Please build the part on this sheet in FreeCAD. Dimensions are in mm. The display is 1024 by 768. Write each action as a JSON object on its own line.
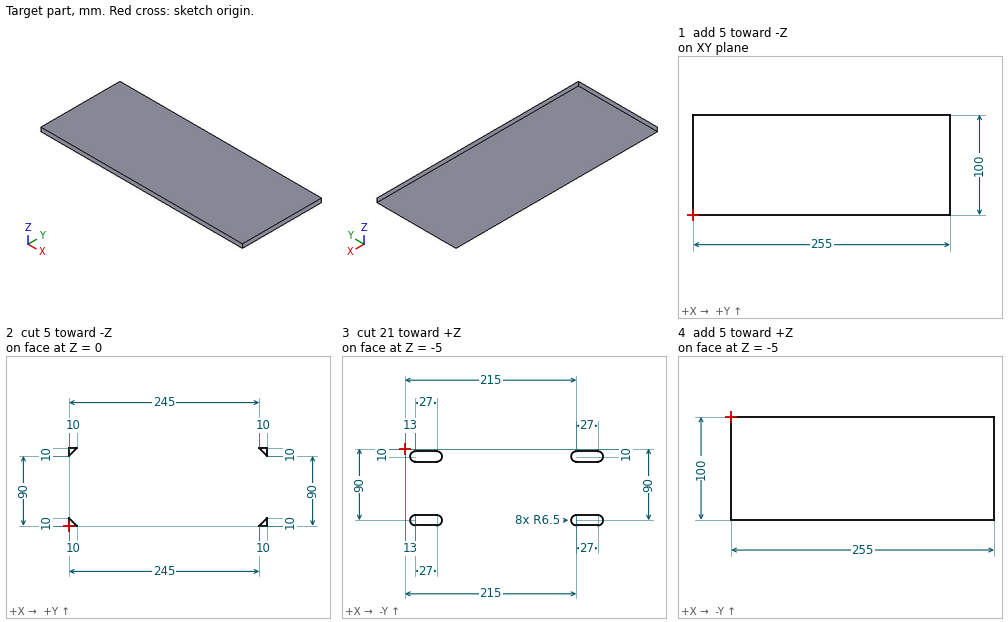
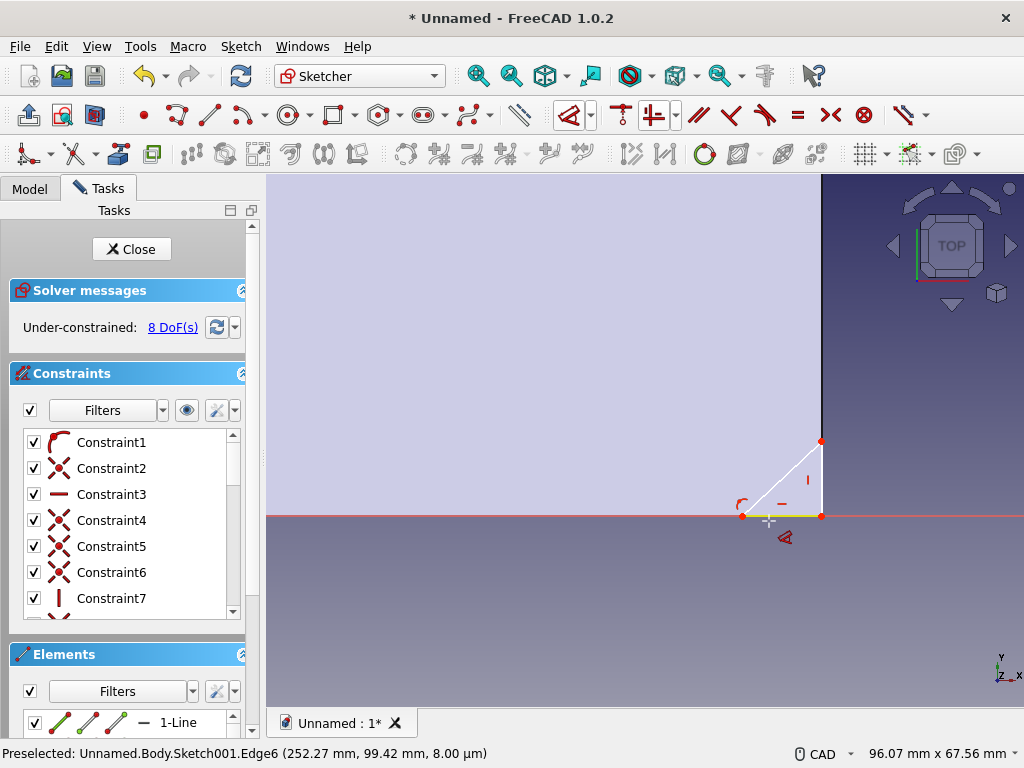
{"action": "left_click", "coordinate": [766, 516]}
{"action": "left_click", "coordinate": [782, 550]}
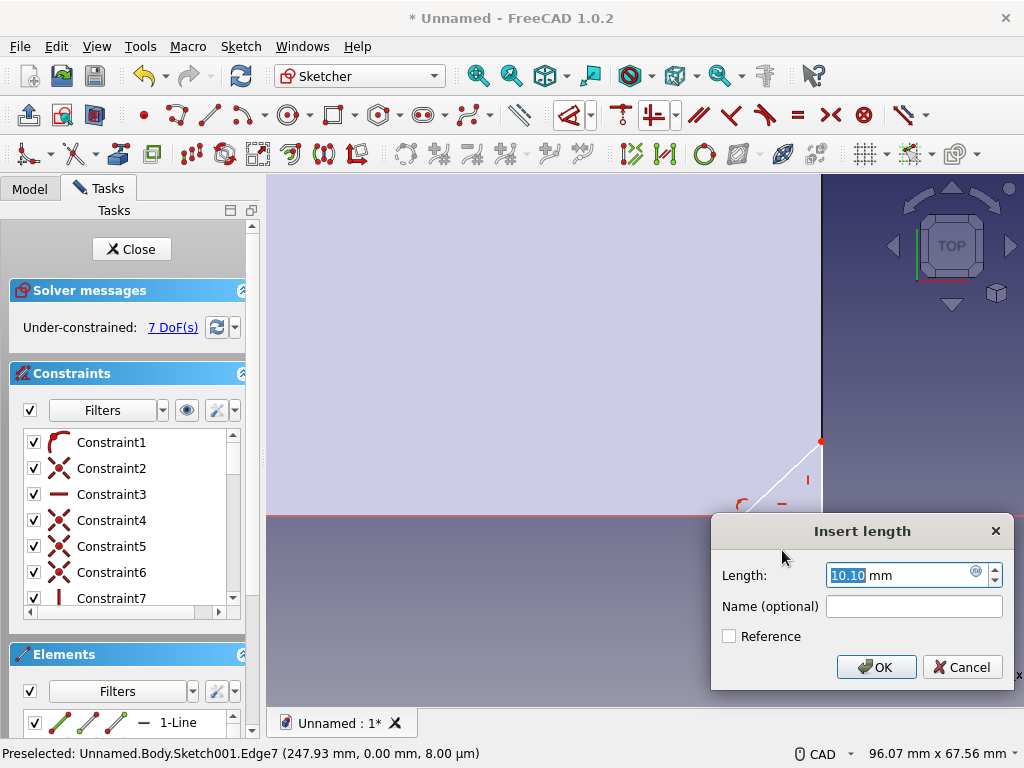
{"action": "type", "text": "10"}
{"action": "key", "text": "Return"}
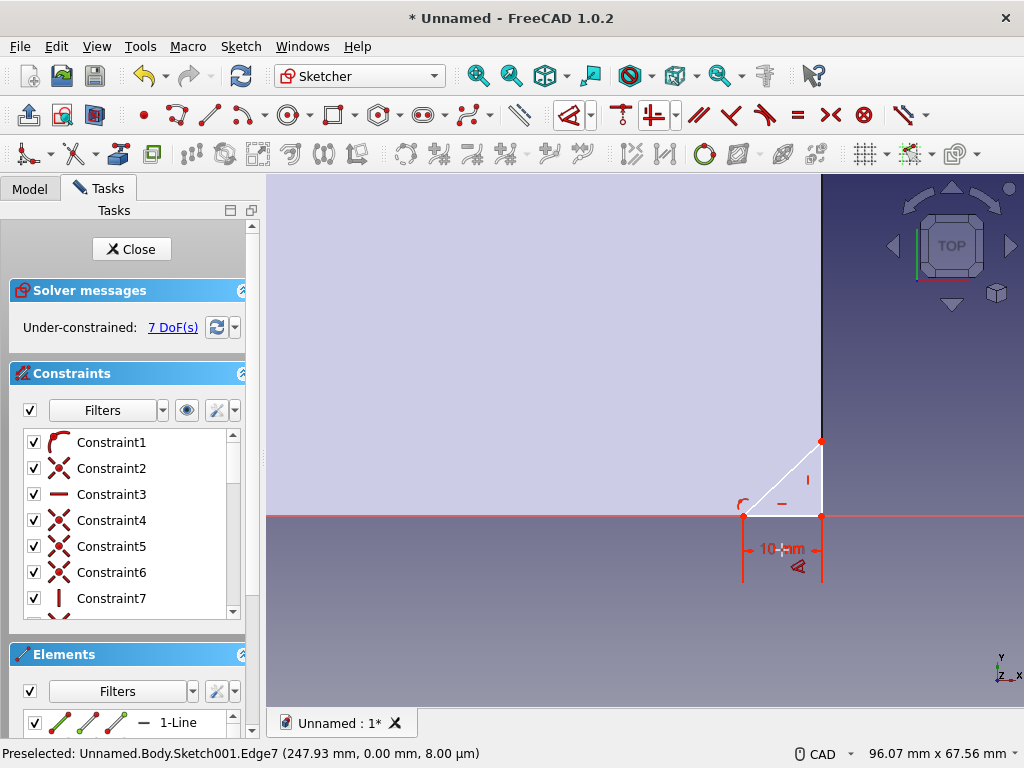
{"action": "left_click", "coordinate": [822, 494]}
{"action": "left_click", "coordinate": [856, 479]}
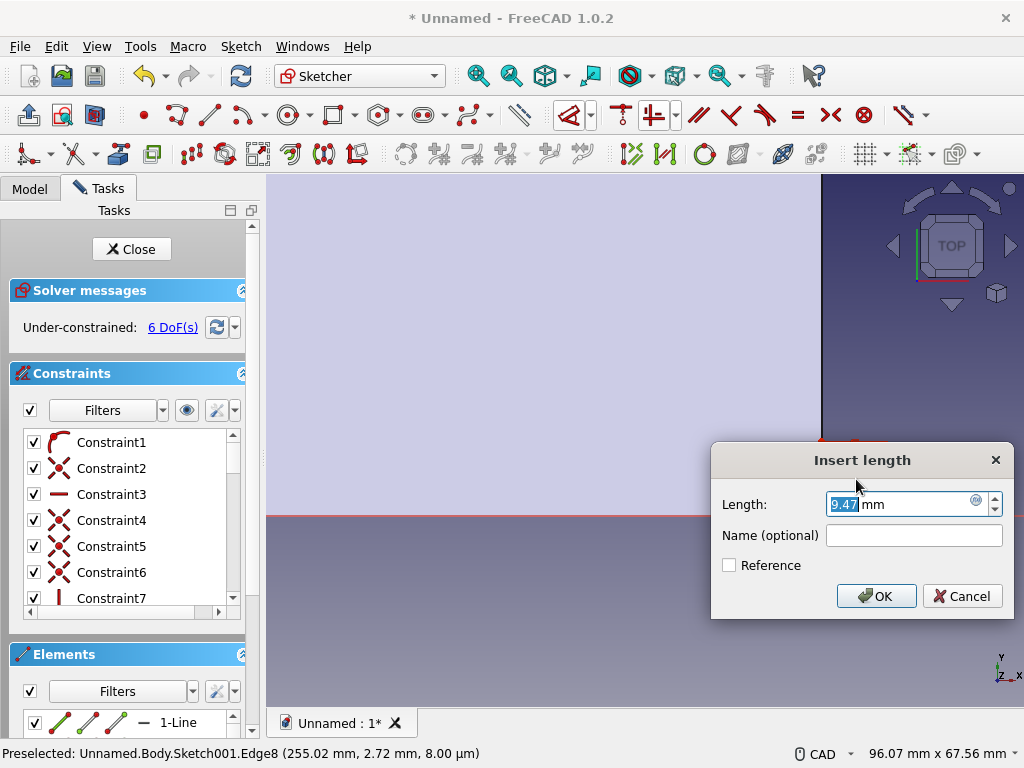
{"action": "type", "text": "10"}
{"action": "key", "text": "Return"}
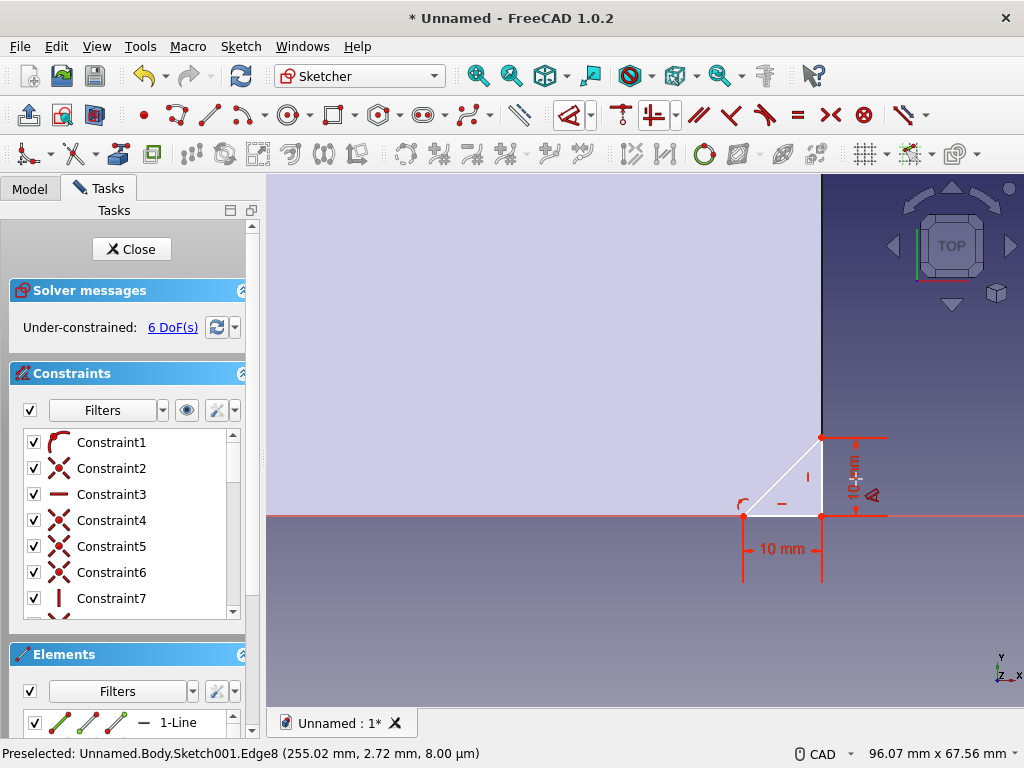
{"action": "scroll", "coordinate": [769, 521], "scroll_direction": "down", "scroll_amount": 8}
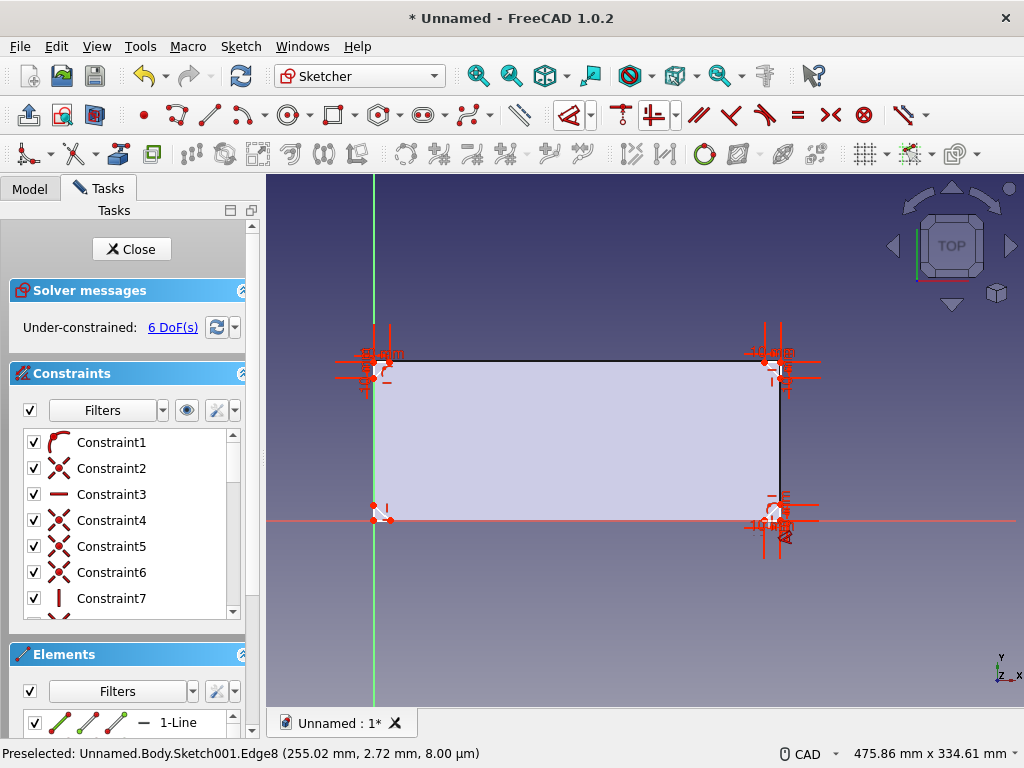
{"action": "scroll", "coordinate": [379, 521], "scroll_direction": "up", "scroll_amount": 6}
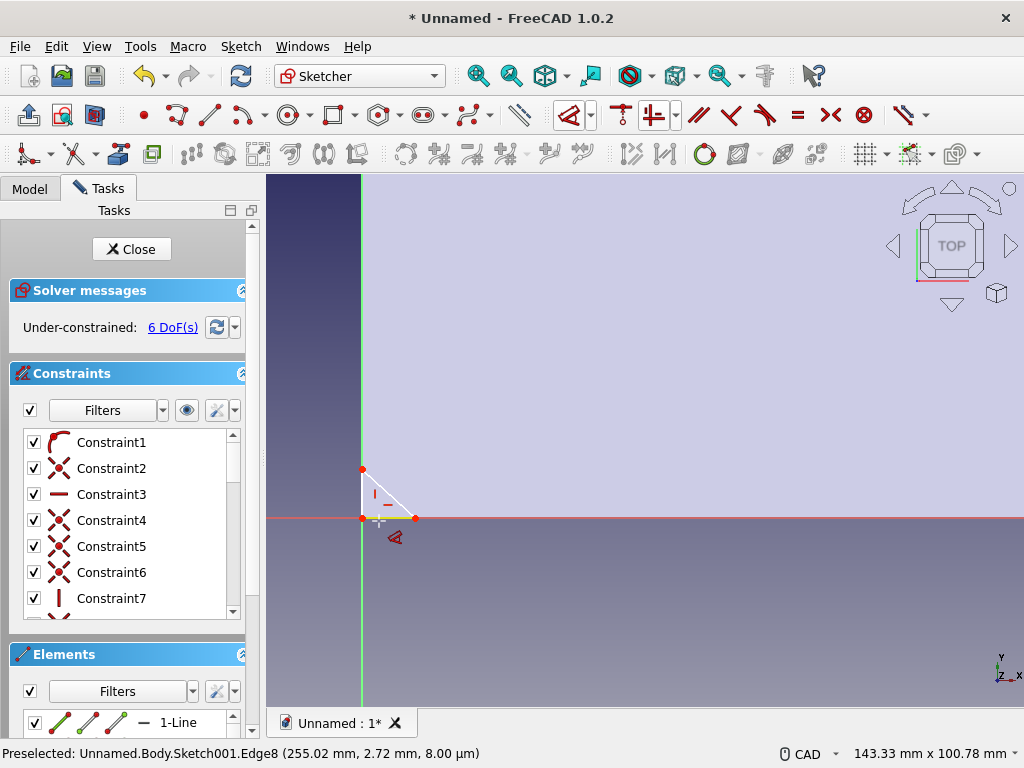
{"action": "left_click", "coordinate": [378, 518]}
{"action": "left_click", "coordinate": [389, 552]}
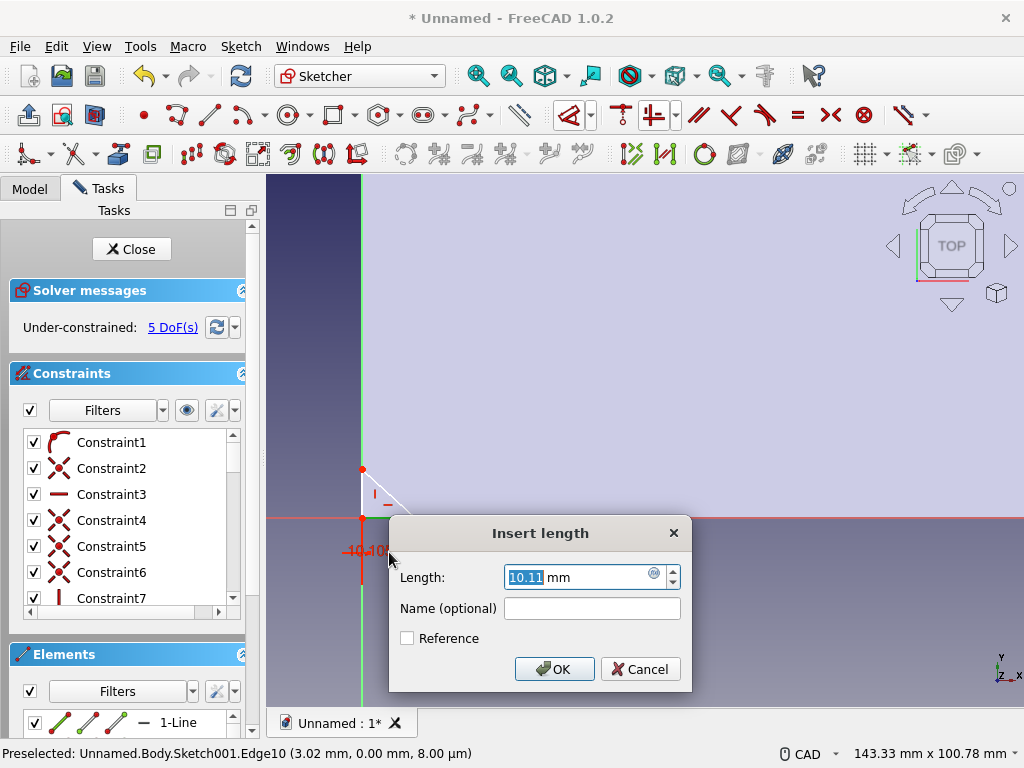
{"action": "type", "text": "10"}
{"action": "key", "text": "Return"}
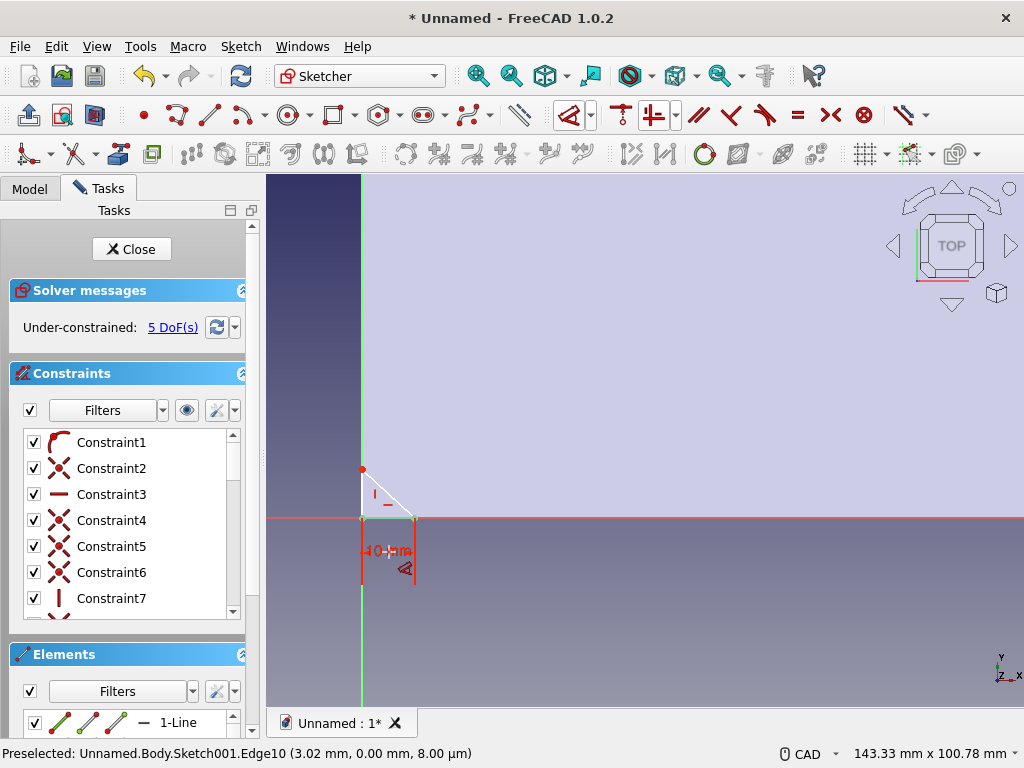
{"action": "scroll", "coordinate": [362, 484], "scroll_direction": "up", "scroll_amount": 2}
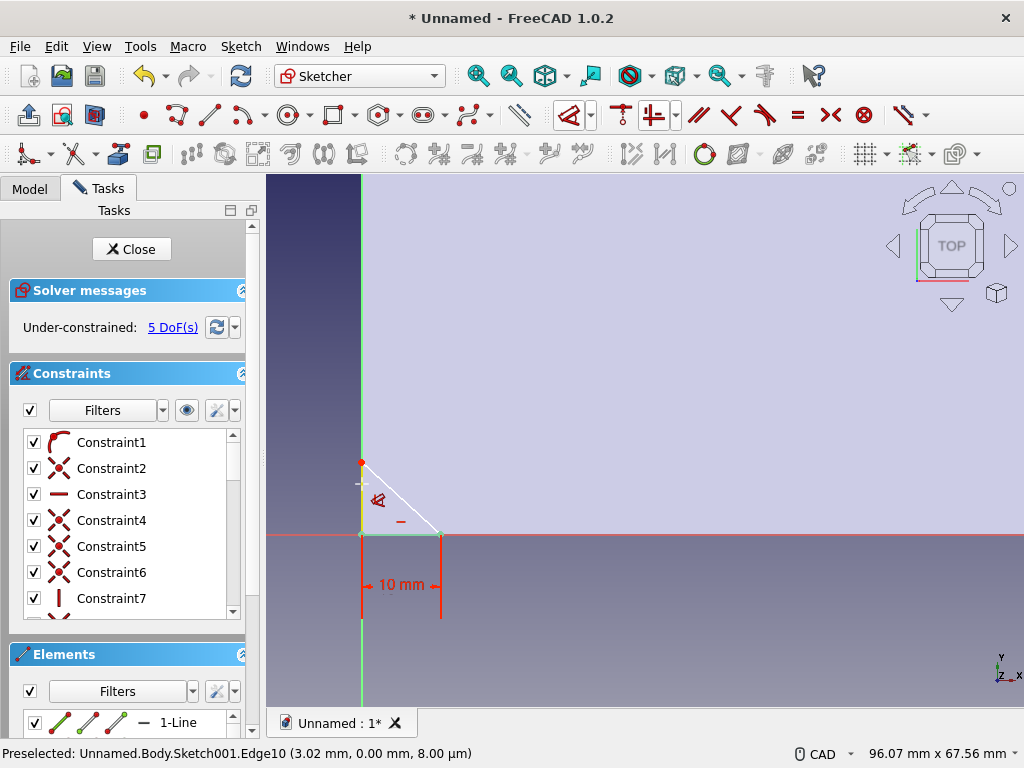
{"action": "left_click", "coordinate": [362, 484]}
{"action": "left_click", "coordinate": [328, 499]}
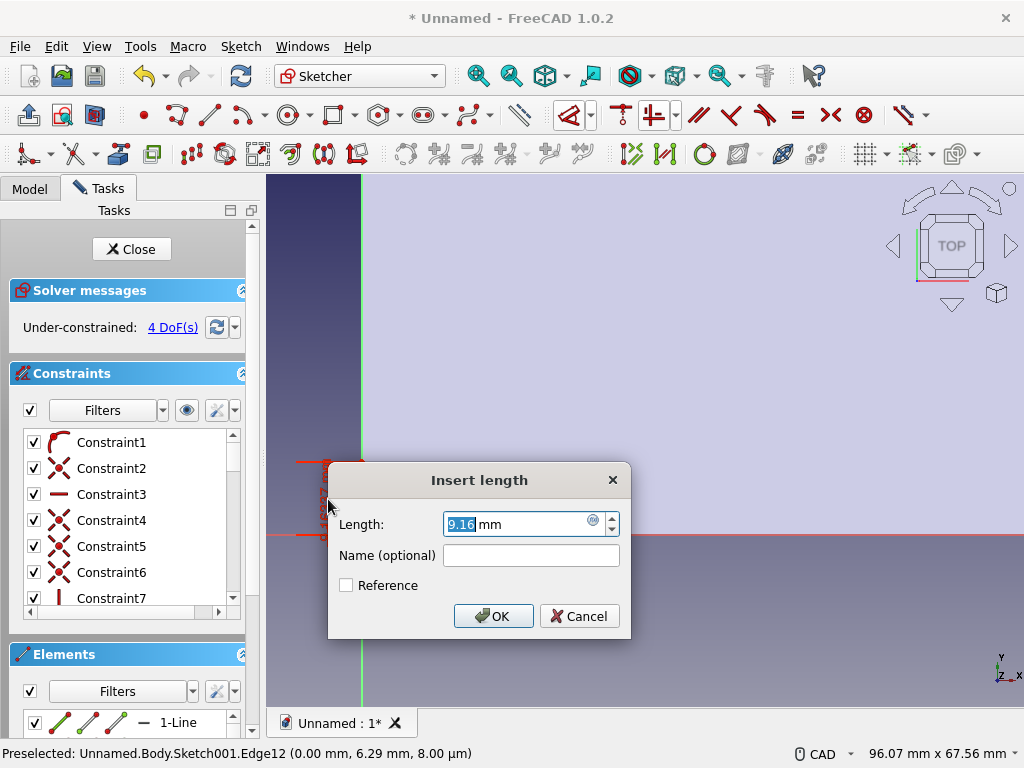
{"action": "type", "text": "10"}
{"action": "key", "text": "Return"}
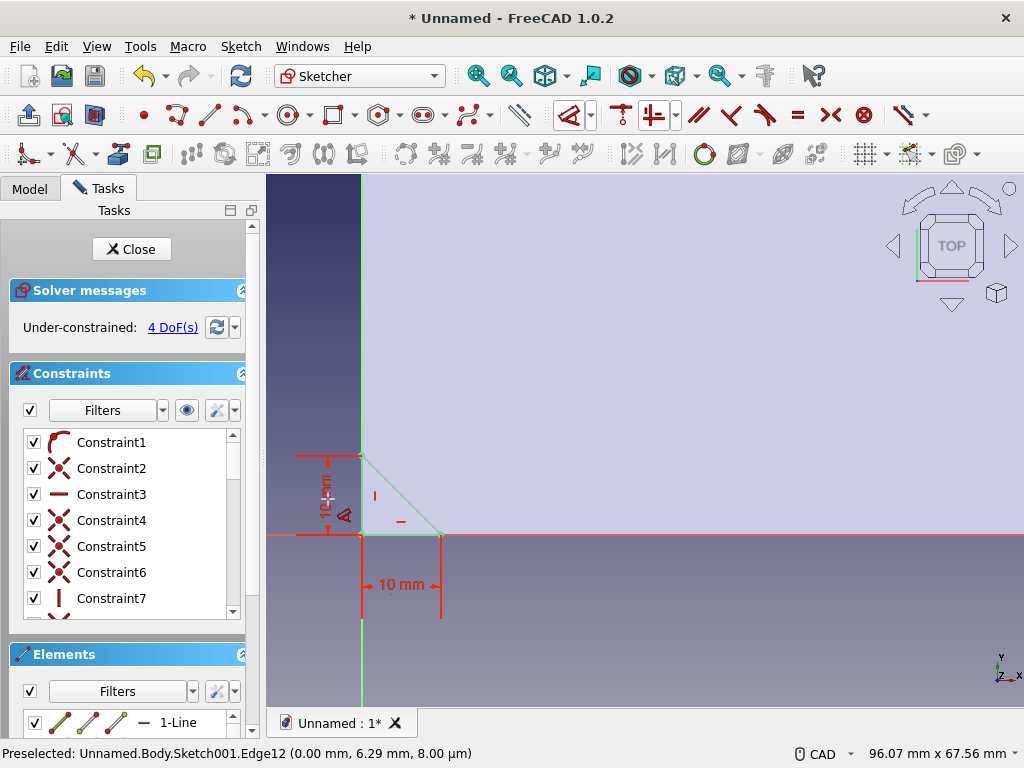
{"action": "scroll", "coordinate": [376, 516], "scroll_direction": "down", "scroll_amount": 8}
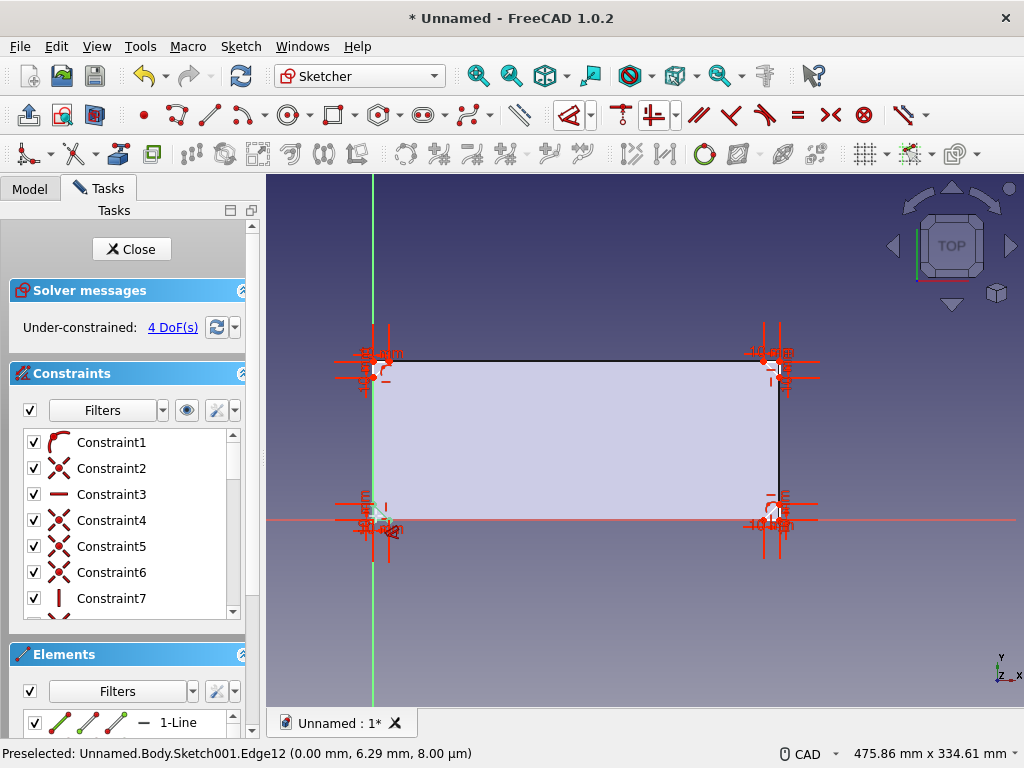
{"action": "left_click", "coordinate": [373, 378]}
{"action": "left_click", "coordinate": [339, 449]}